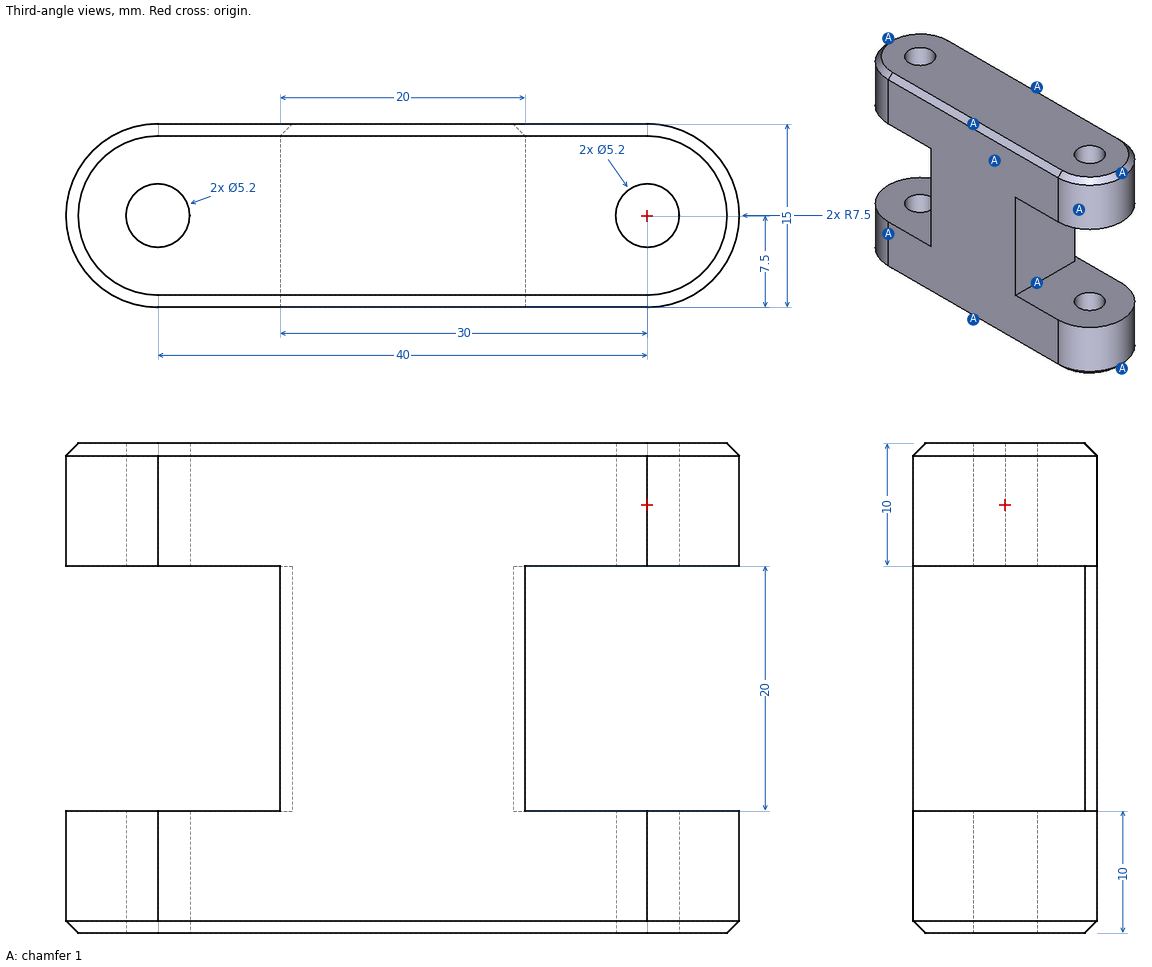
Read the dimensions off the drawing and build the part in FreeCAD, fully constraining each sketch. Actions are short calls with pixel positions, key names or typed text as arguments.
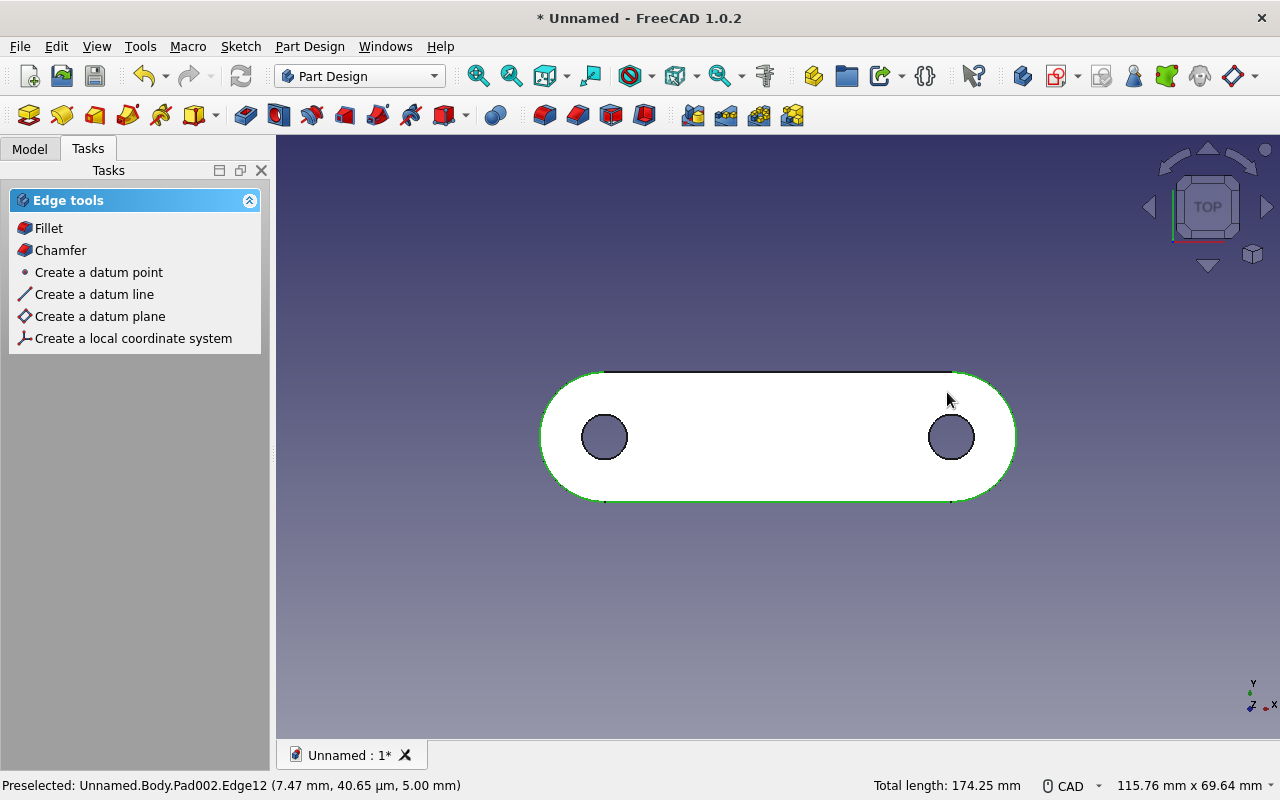
click(778, 371, ctrl)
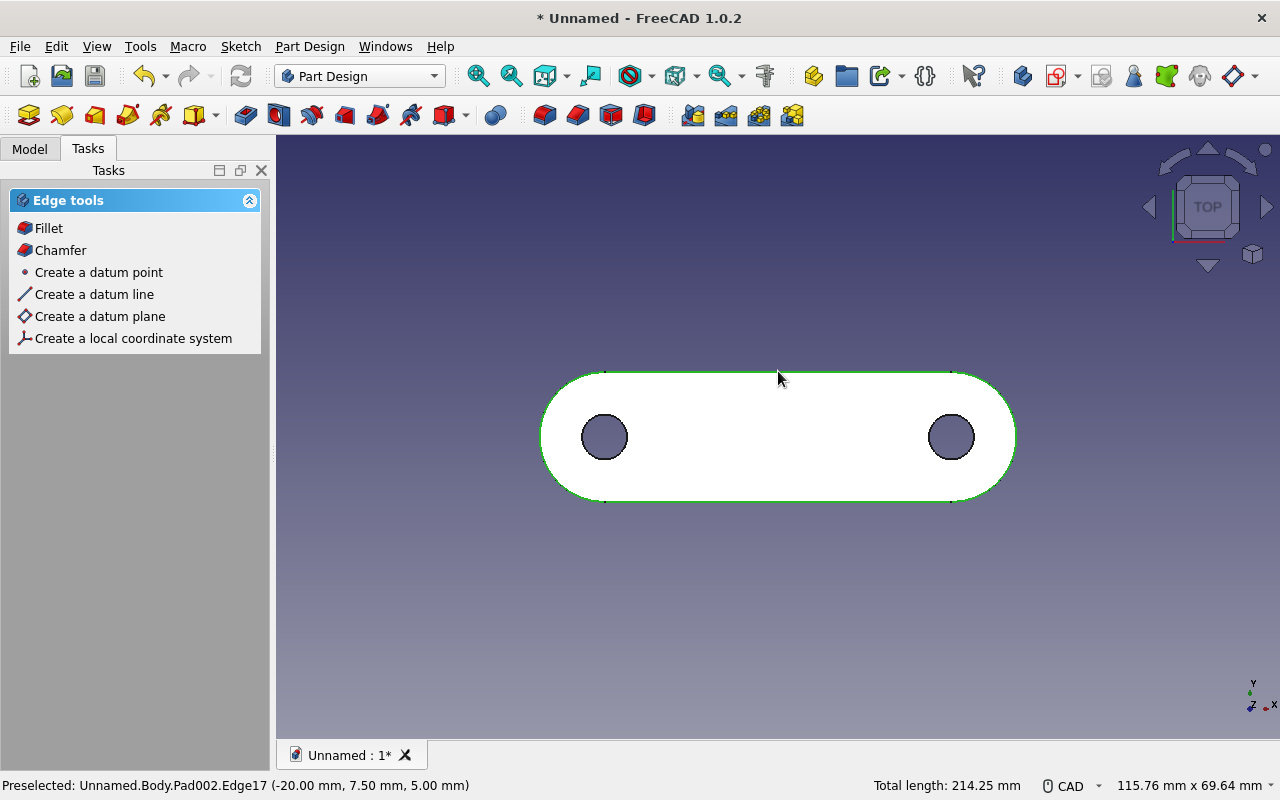
key(1)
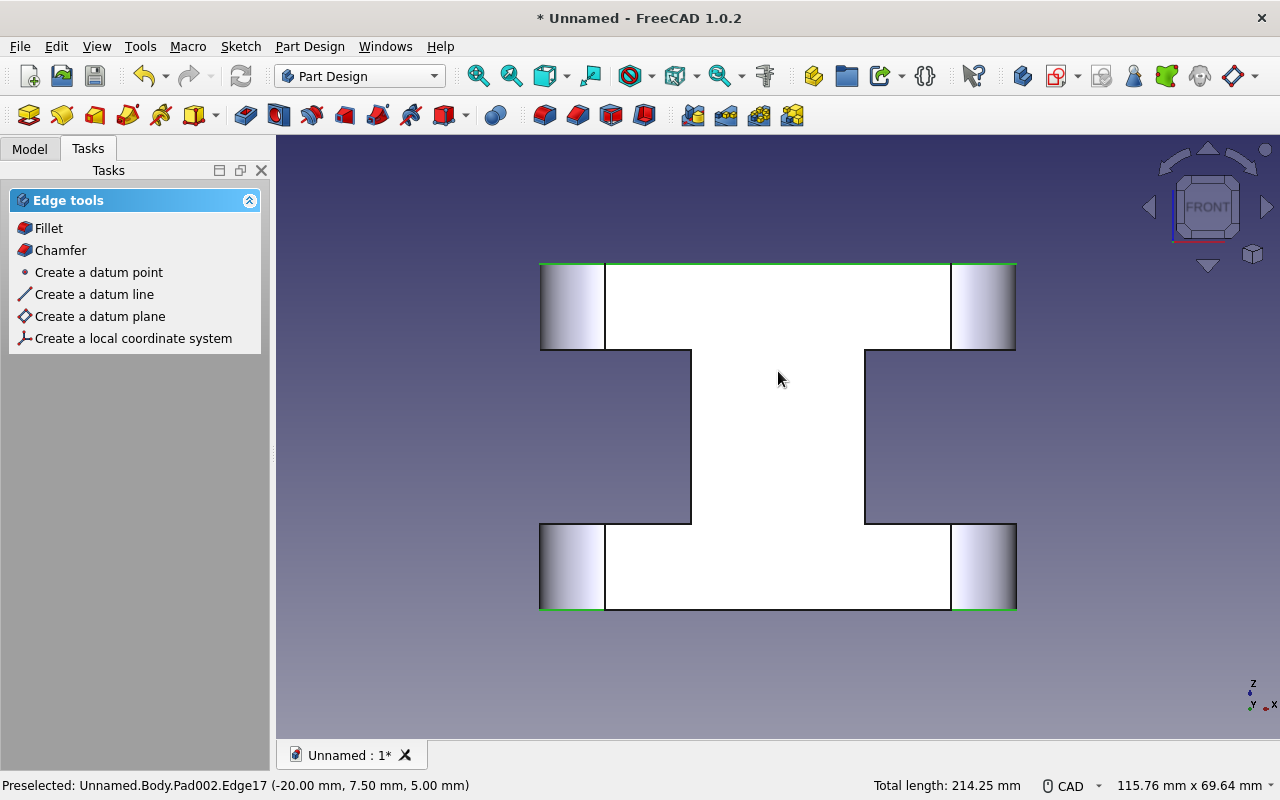
click(778, 609, ctrl)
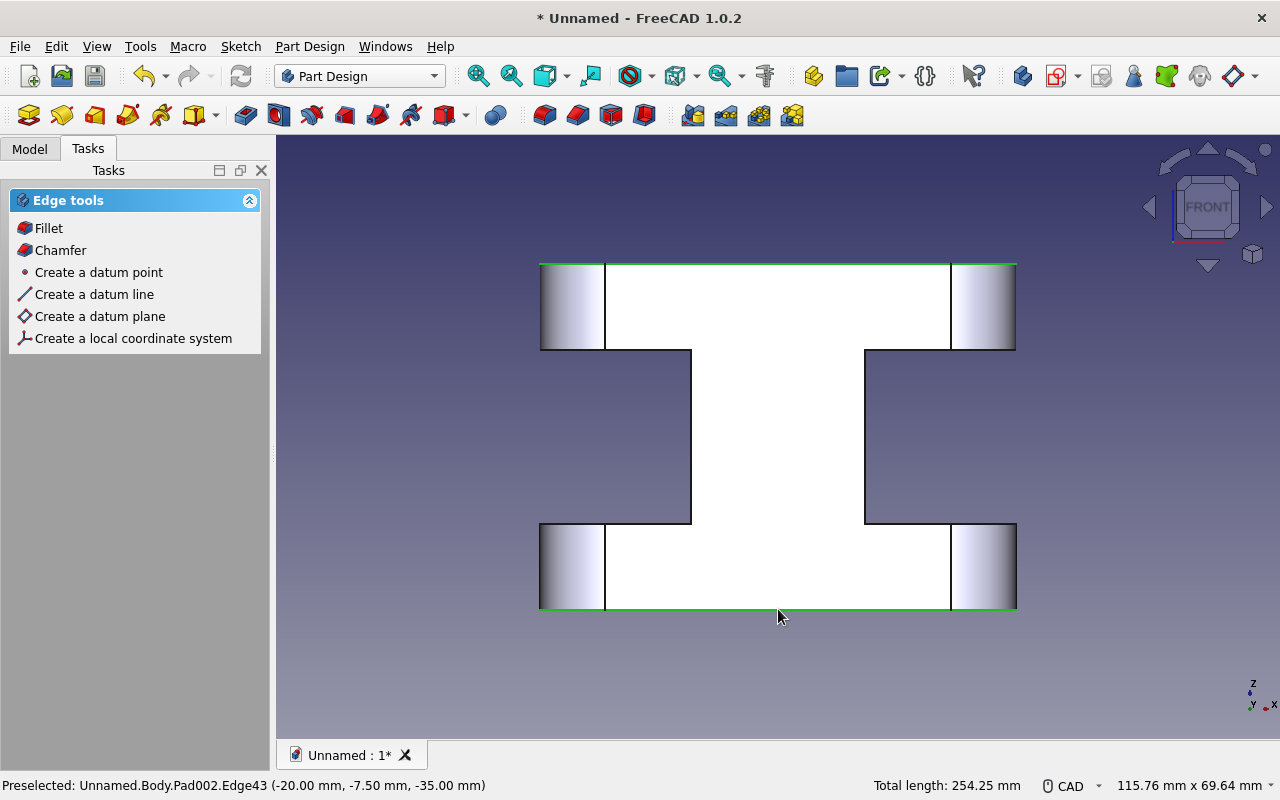
key(3)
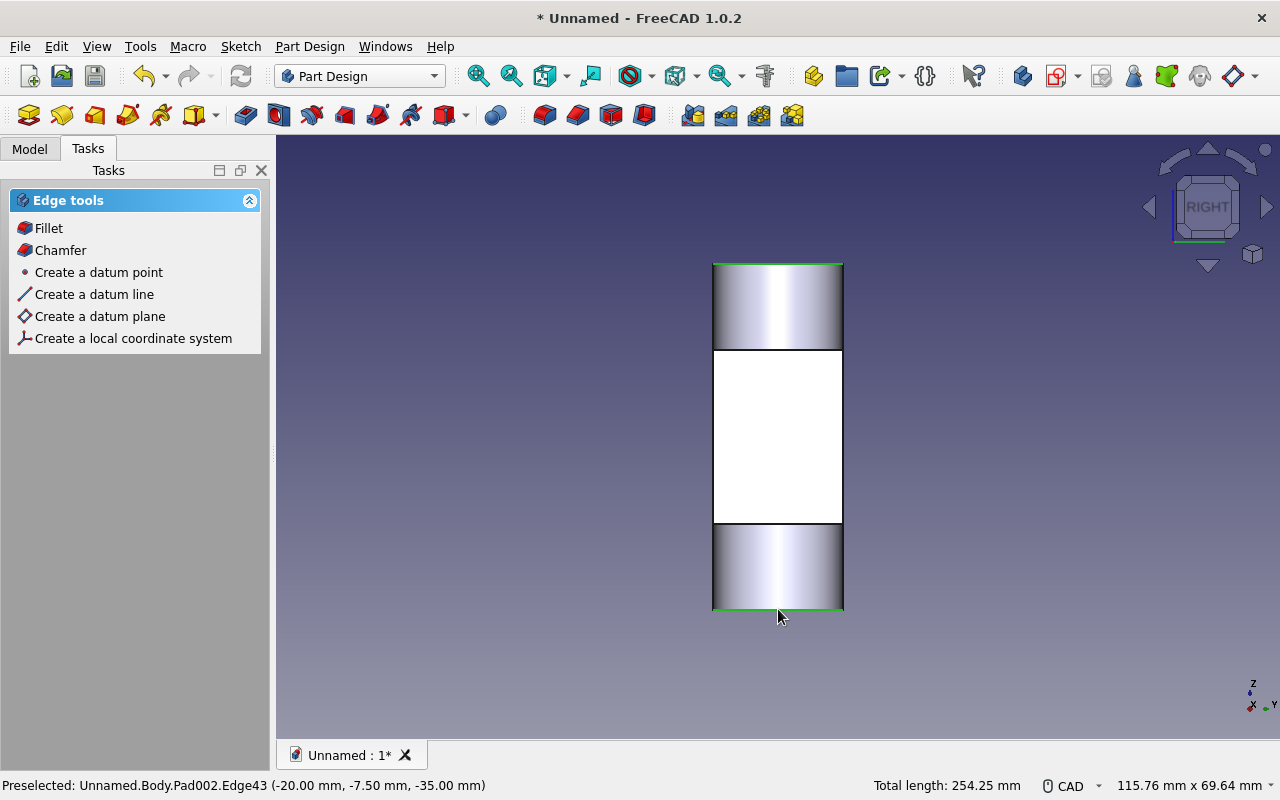
click(843, 436, ctrl)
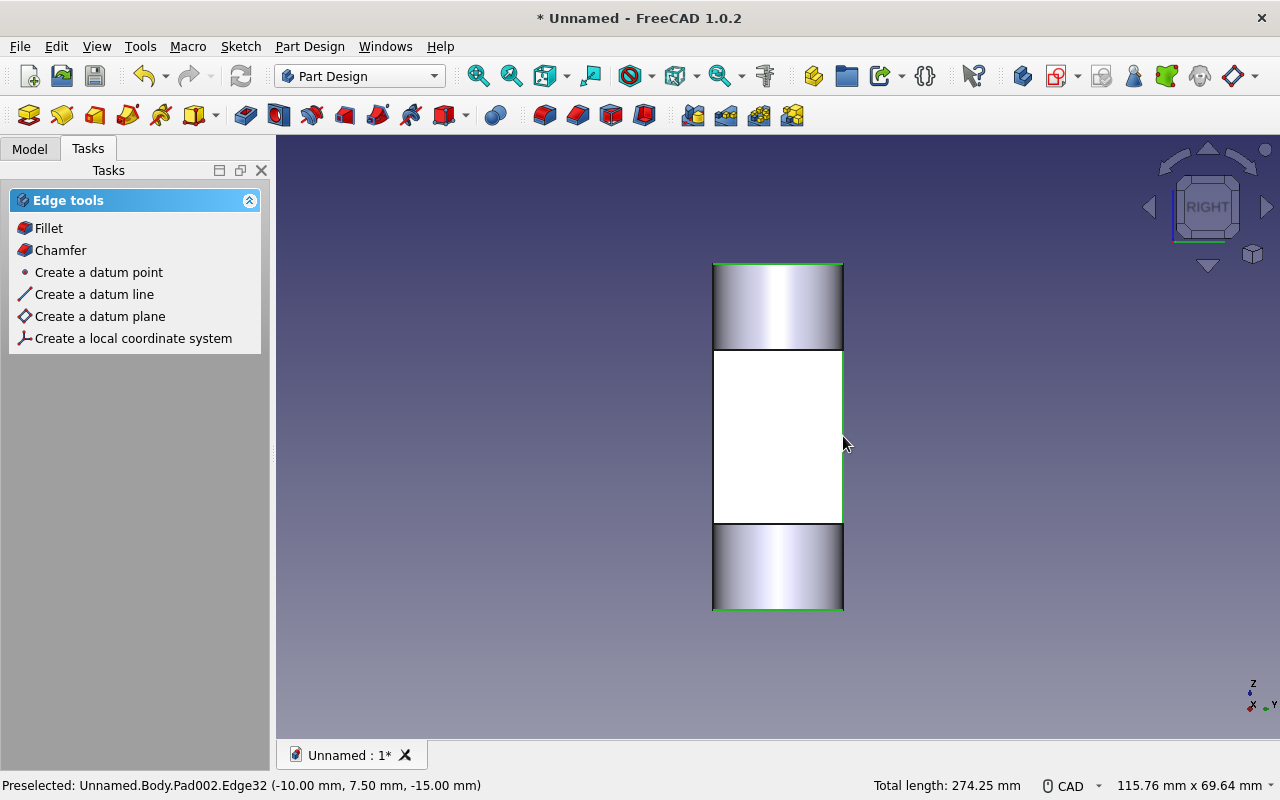
key(5)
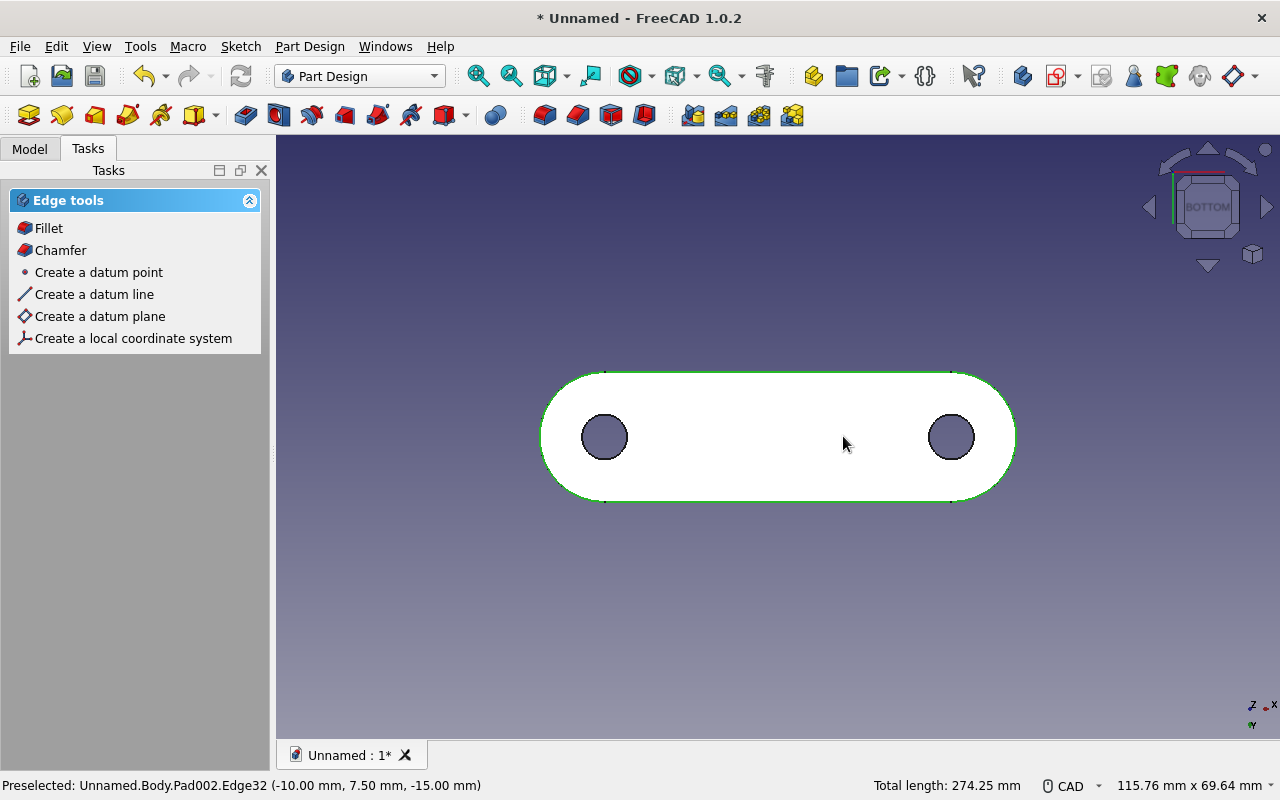
key(4)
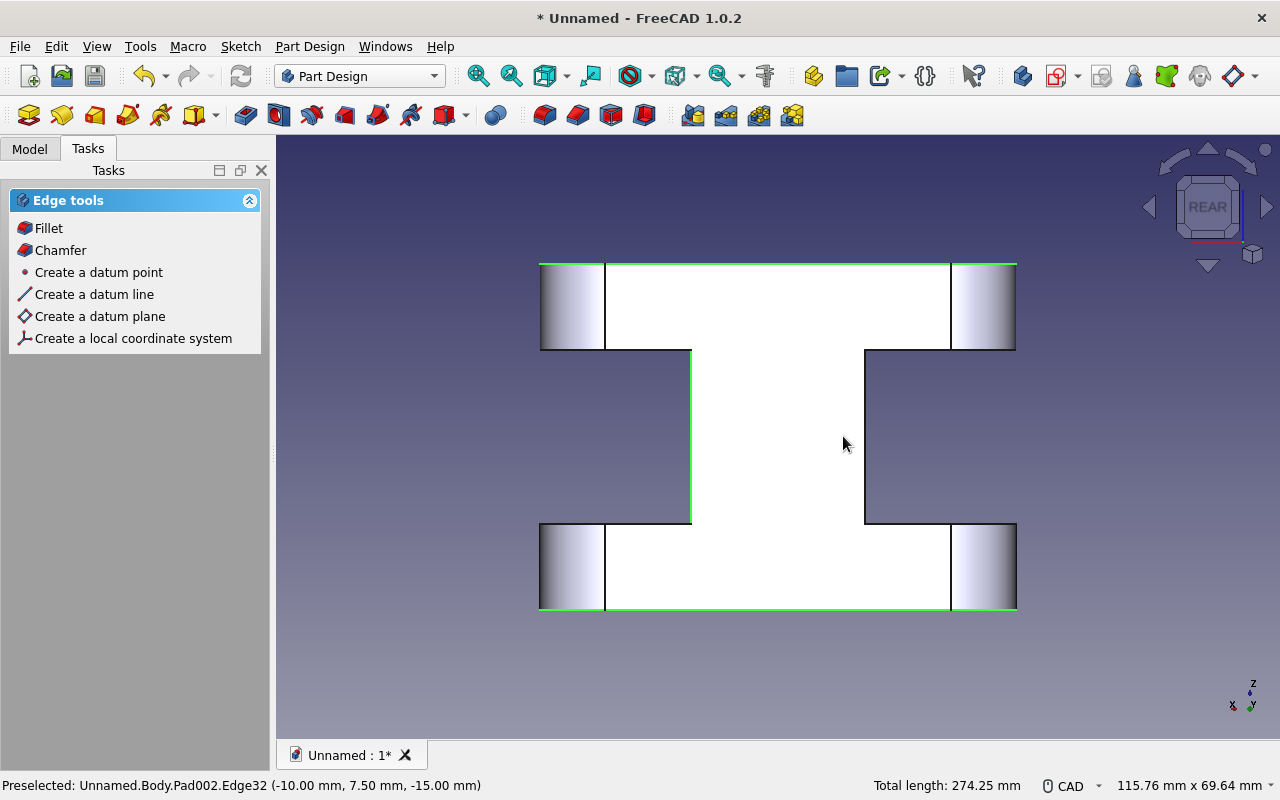
click(865, 436, ctrl)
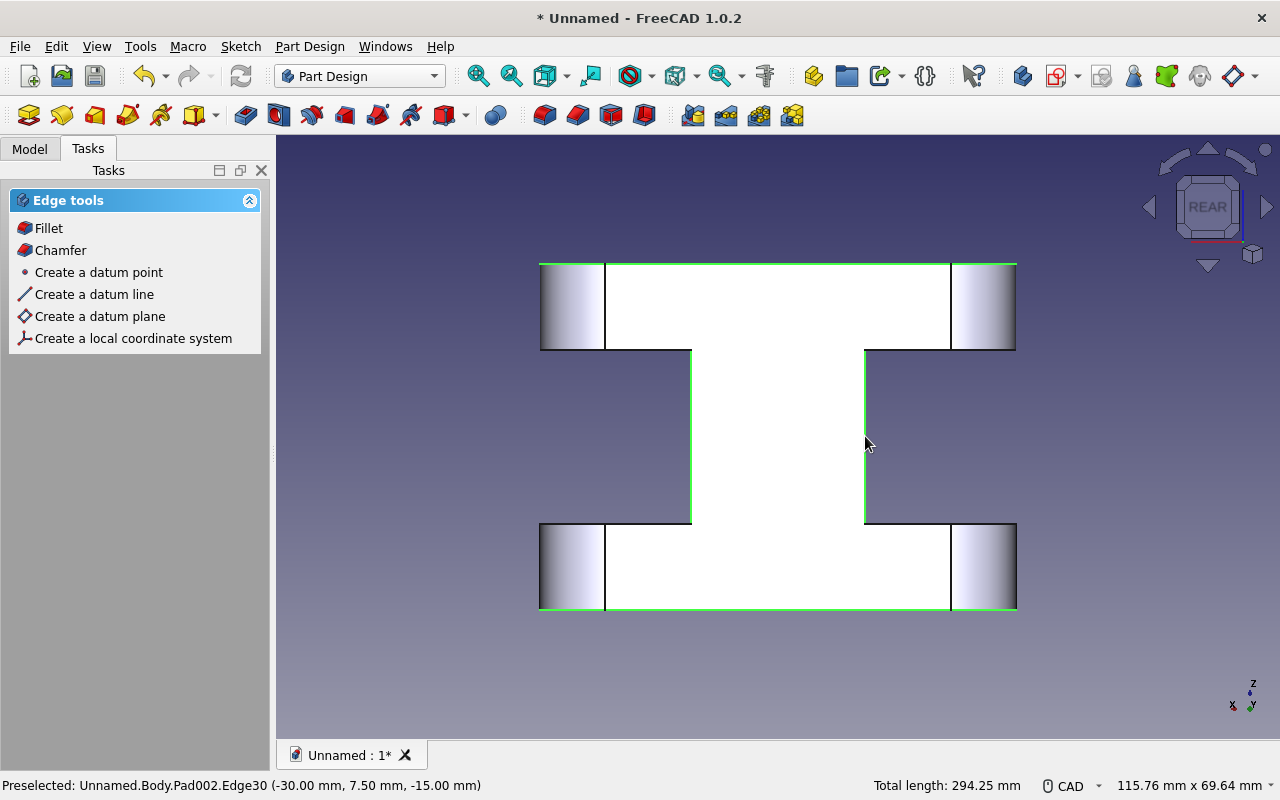
click(578, 116)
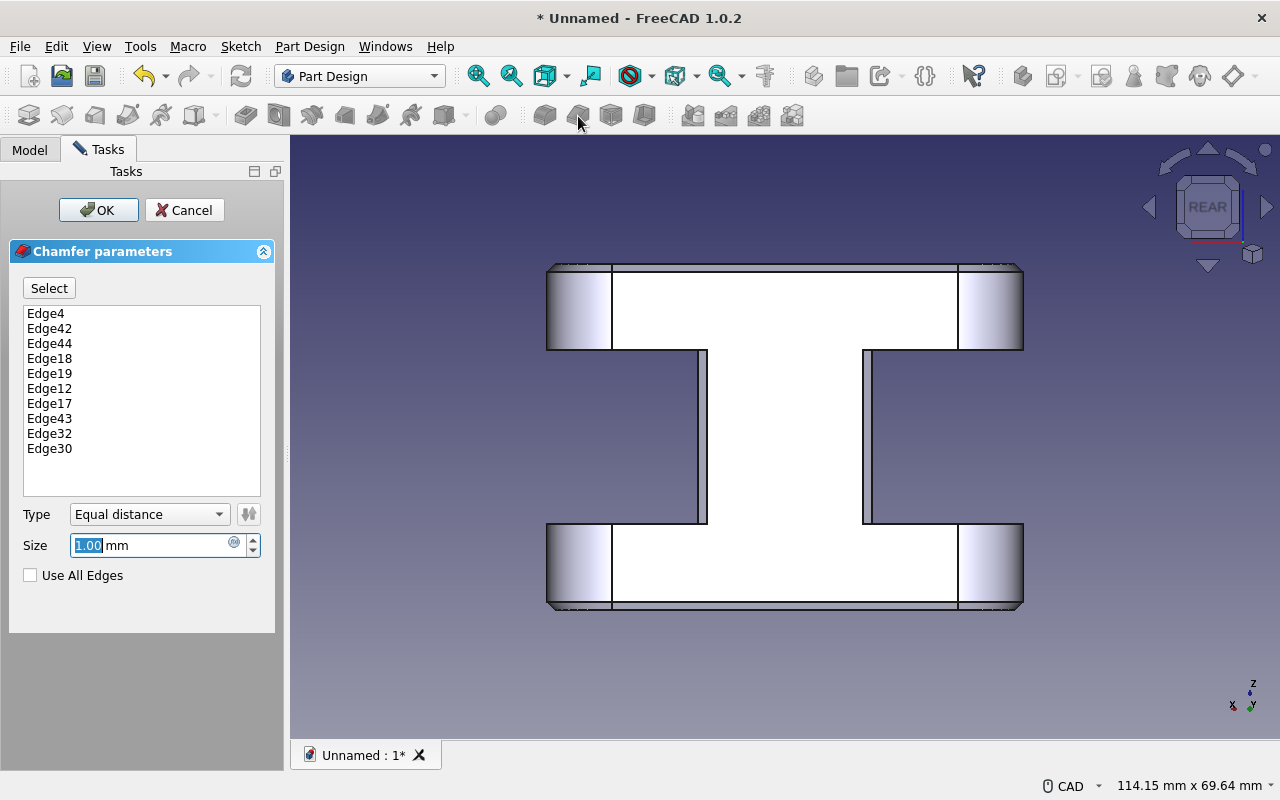
text(1)
key(Tab)